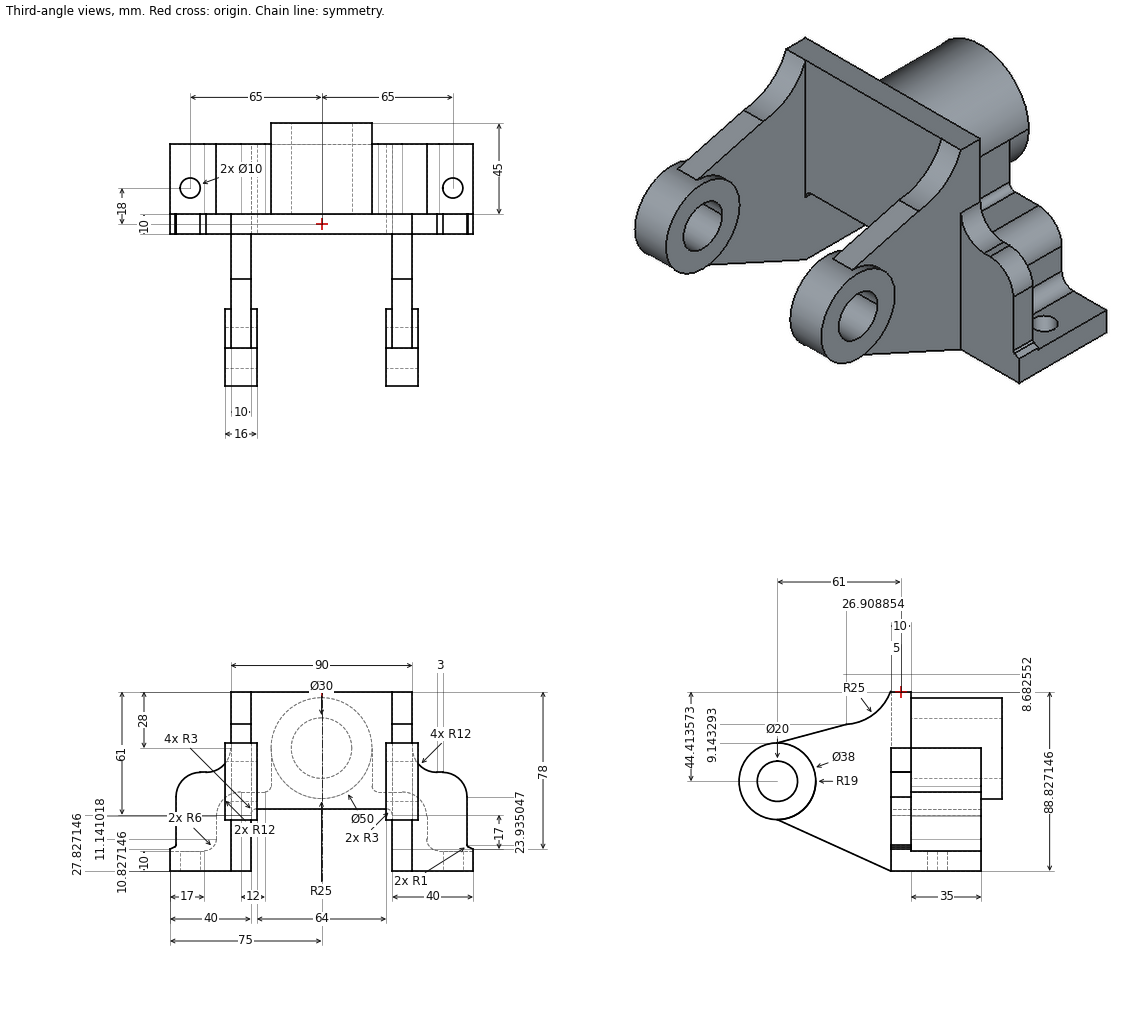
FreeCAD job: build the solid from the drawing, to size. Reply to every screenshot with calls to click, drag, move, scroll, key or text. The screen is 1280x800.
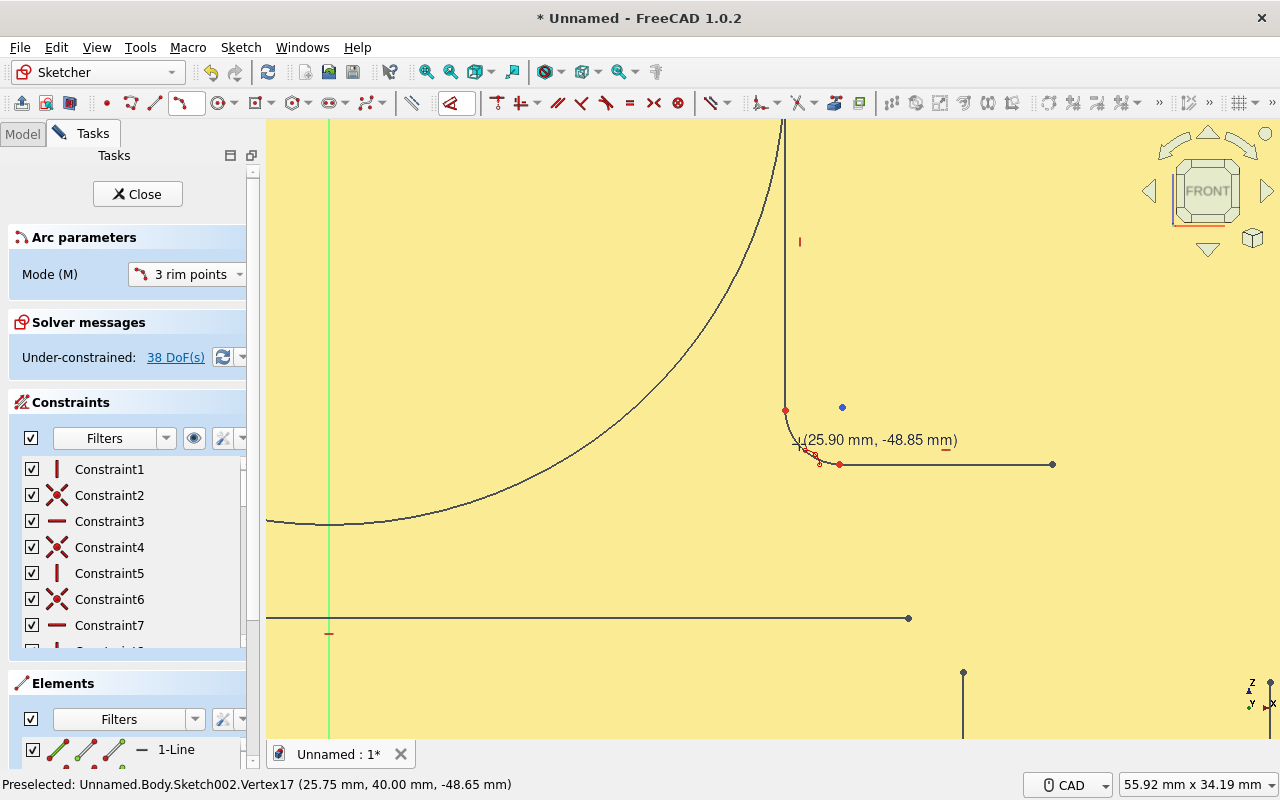
scroll(799, 445, down, 8)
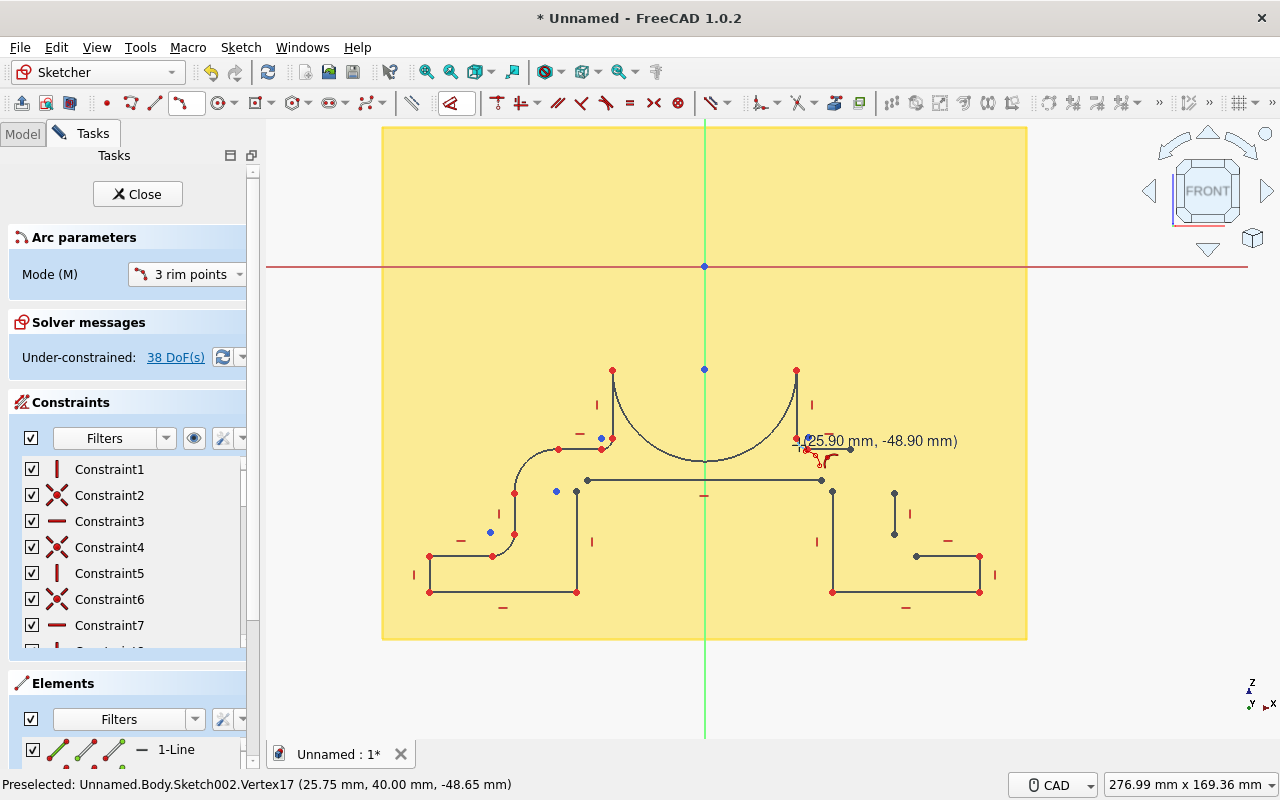
click(851, 449)
click(895, 493)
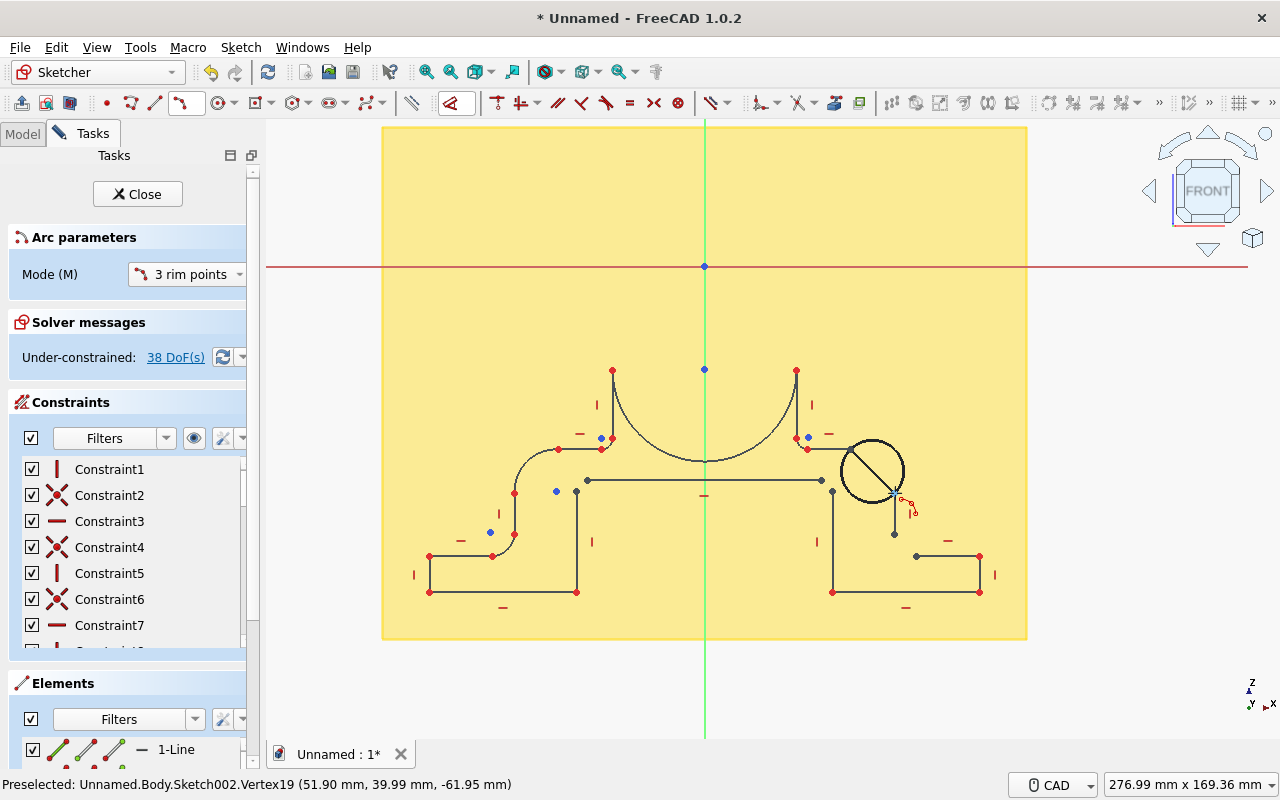
scroll(882, 461, up, 2)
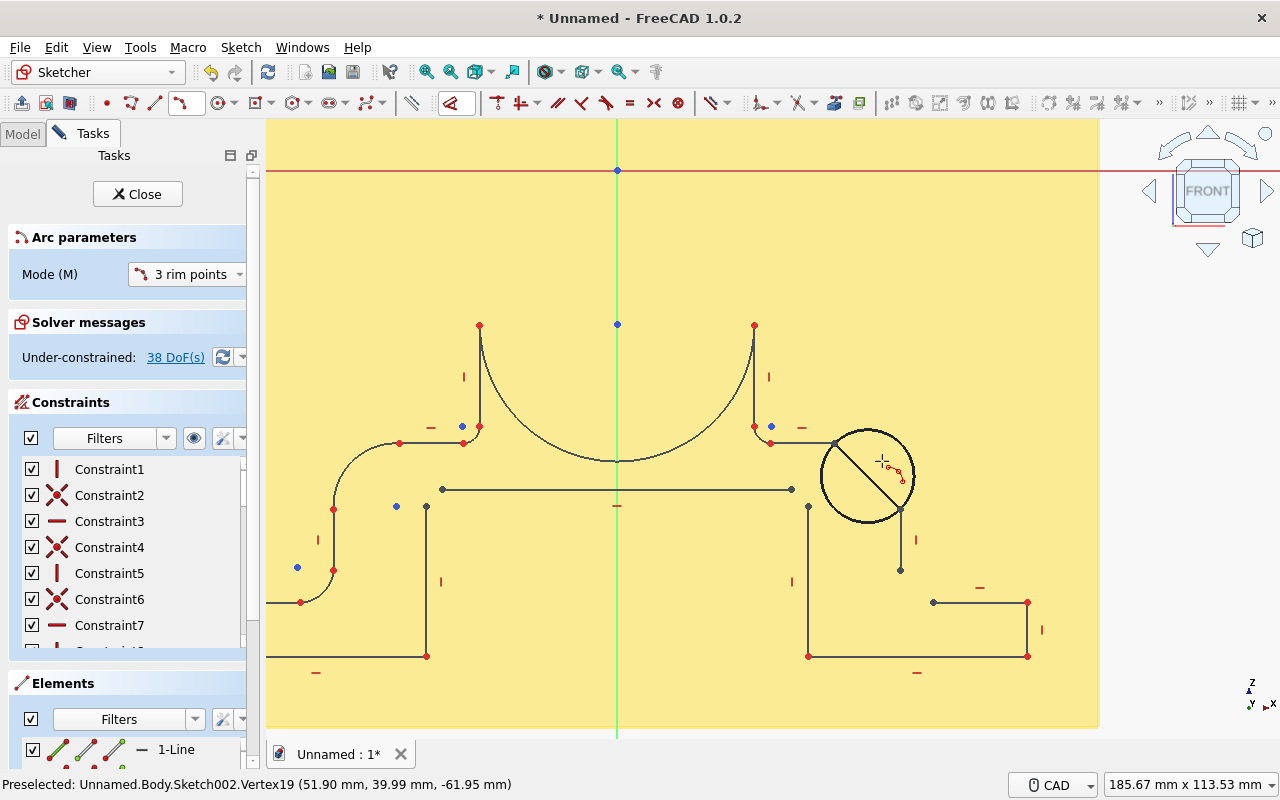
click(882, 461)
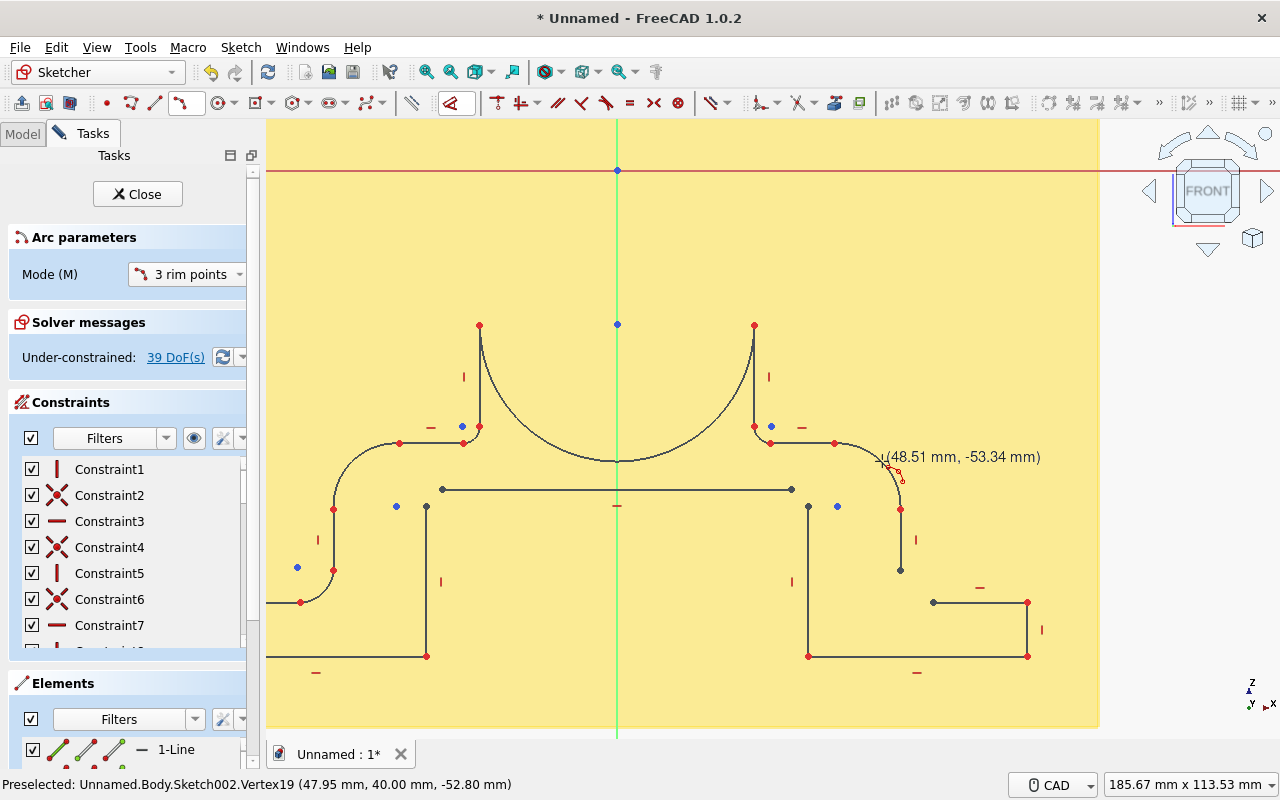
click(901, 570)
click(933, 603)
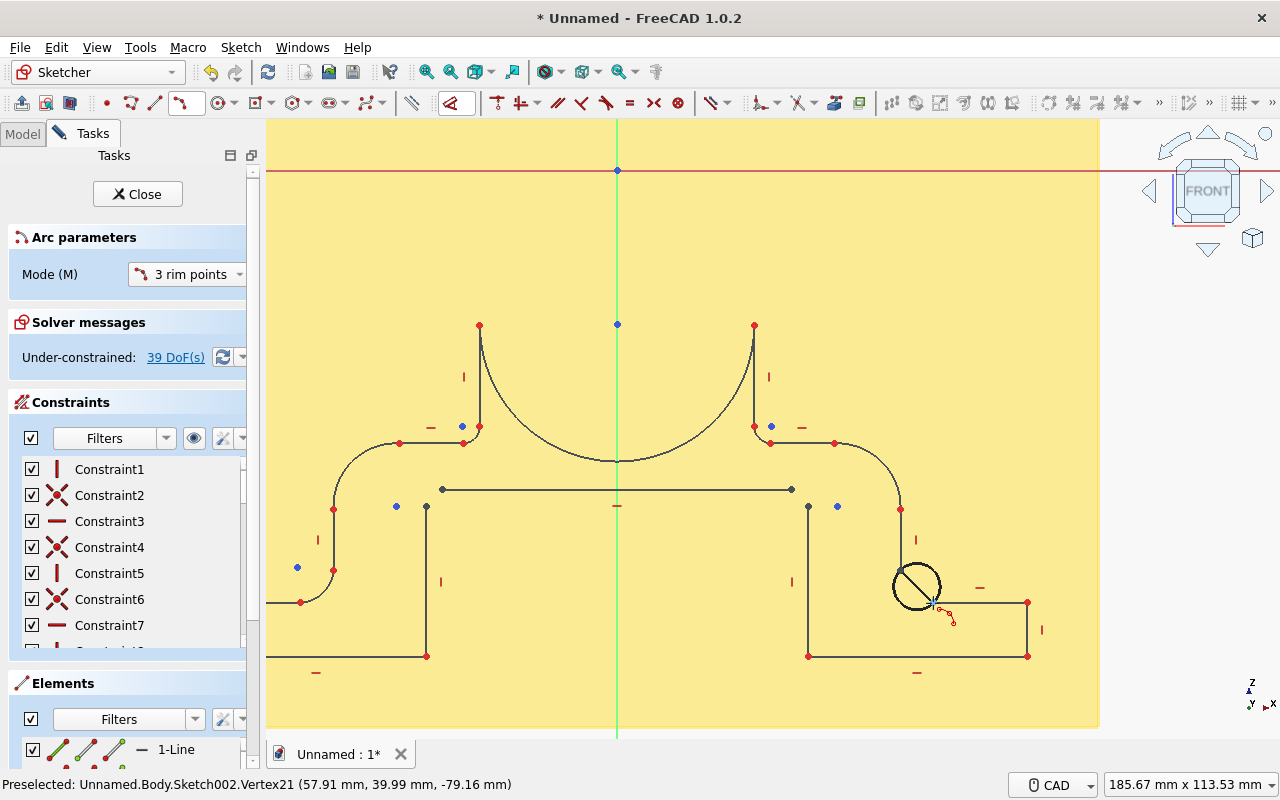
scroll(911, 592, up, 3)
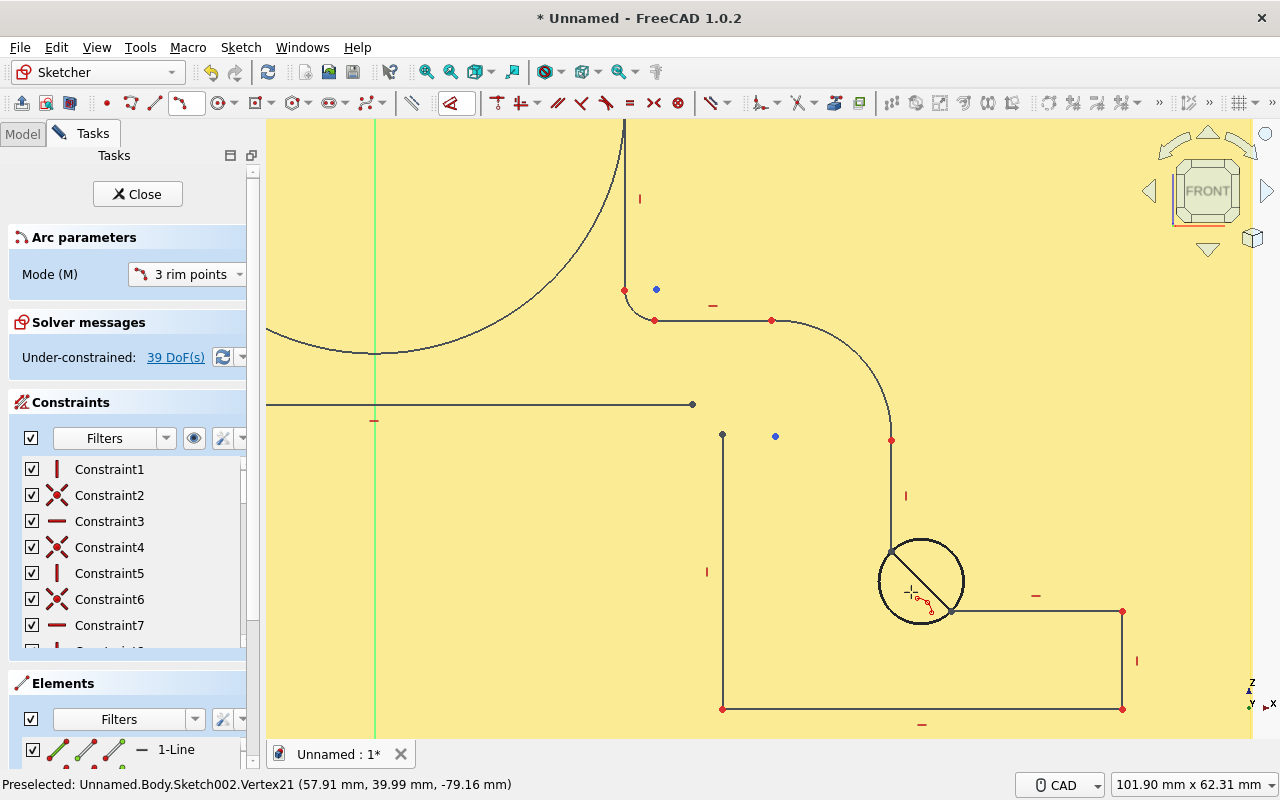
click(910, 591)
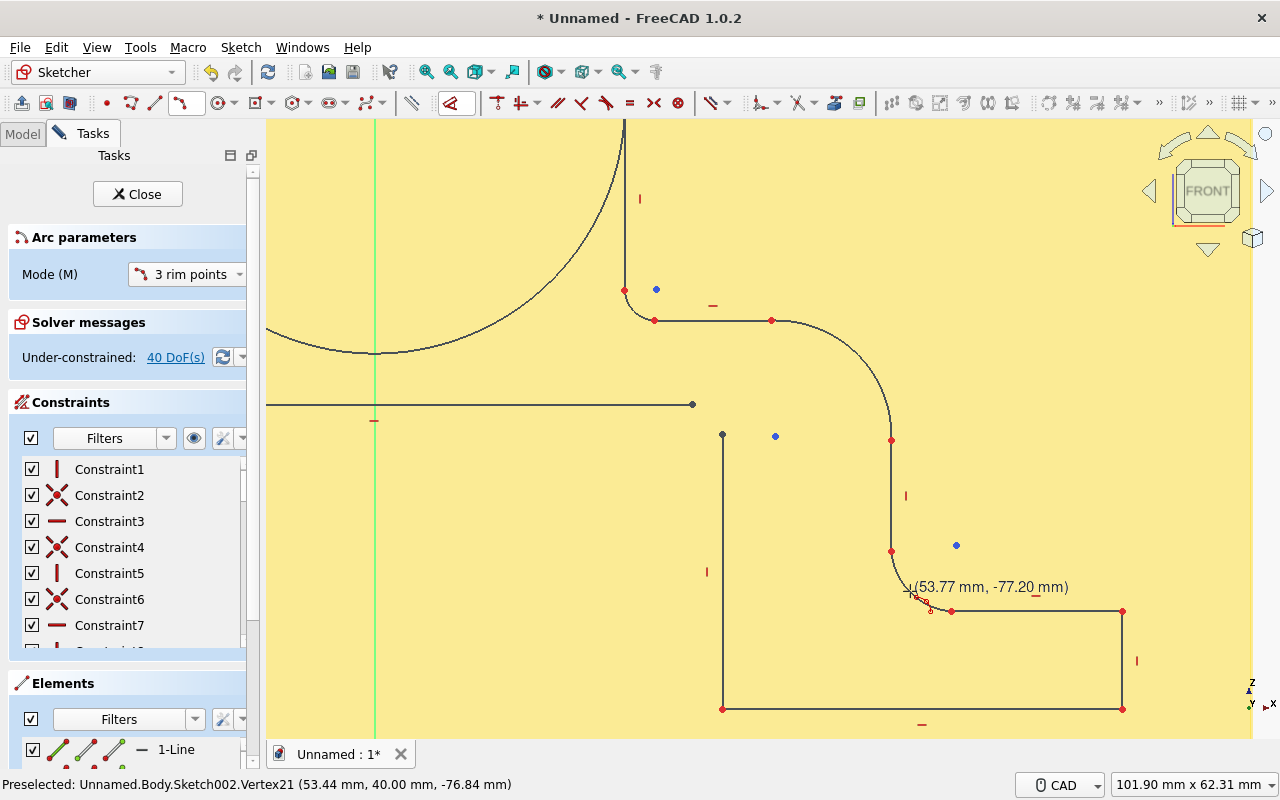
click(723, 435)
click(693, 405)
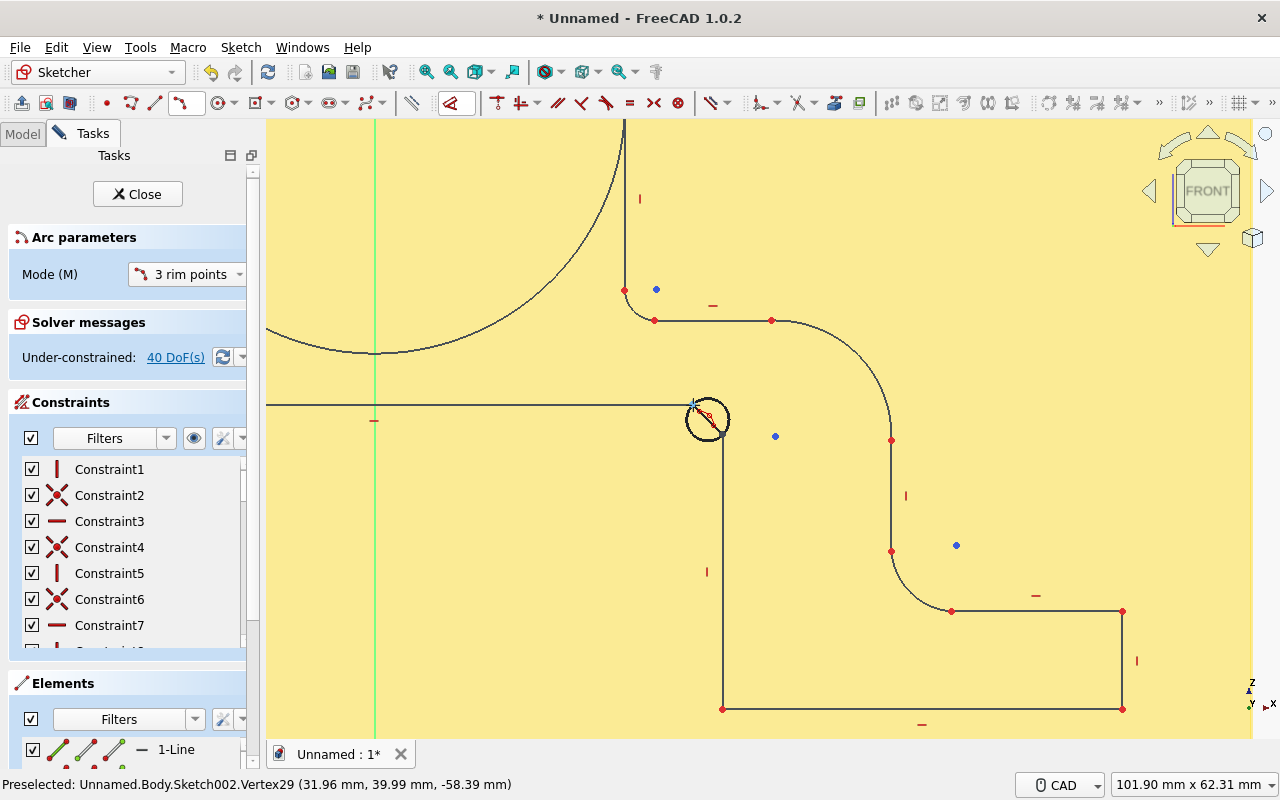
scroll(714, 410, up, 3)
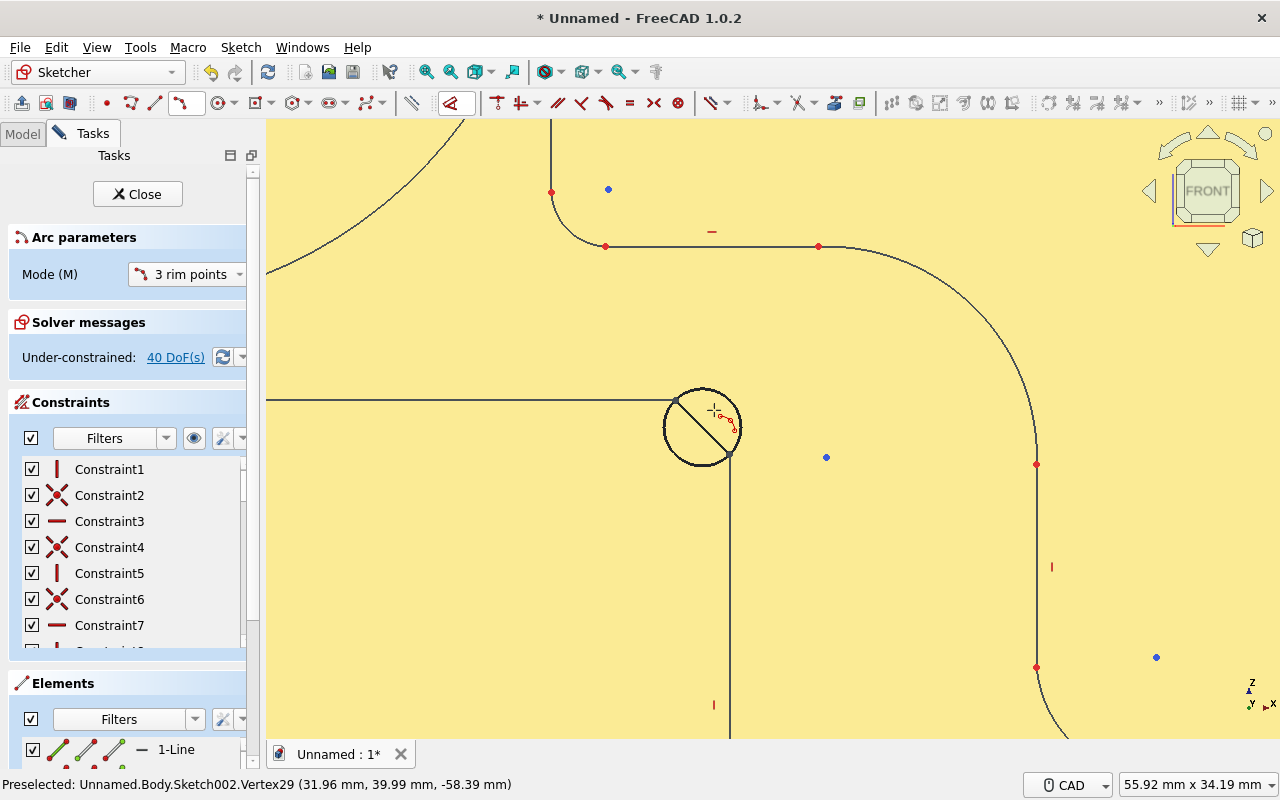
click(714, 409)